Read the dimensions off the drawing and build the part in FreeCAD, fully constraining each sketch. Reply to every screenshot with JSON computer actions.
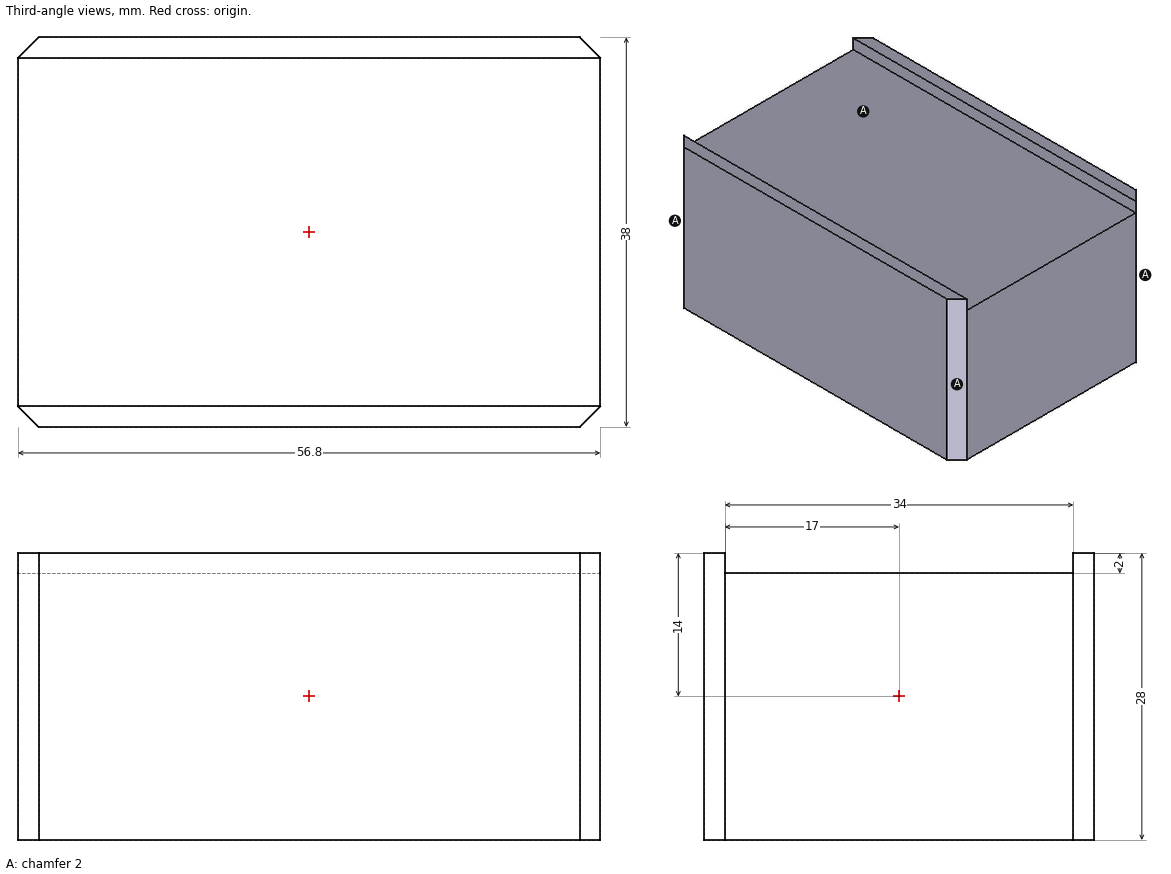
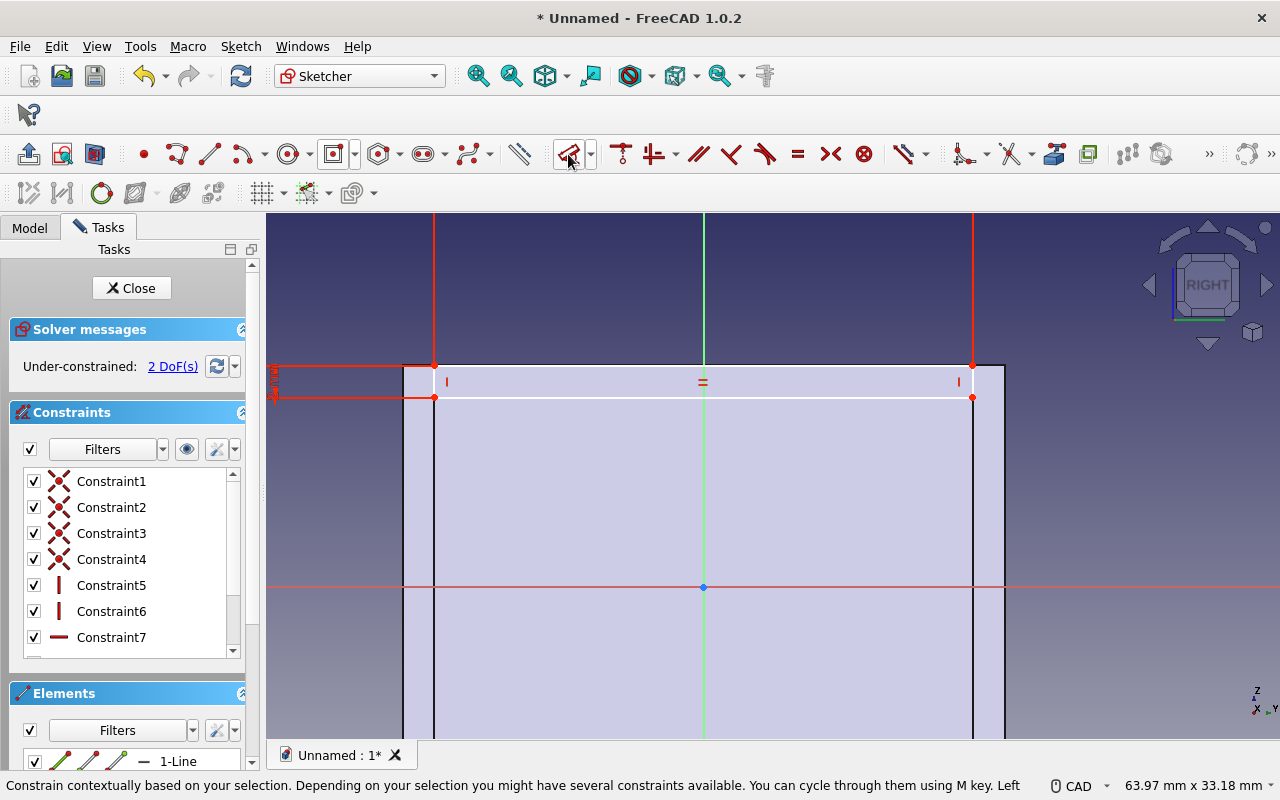
{"action": "left_click", "coordinate": [434, 366]}
{"action": "left_click", "coordinate": [569, 621]}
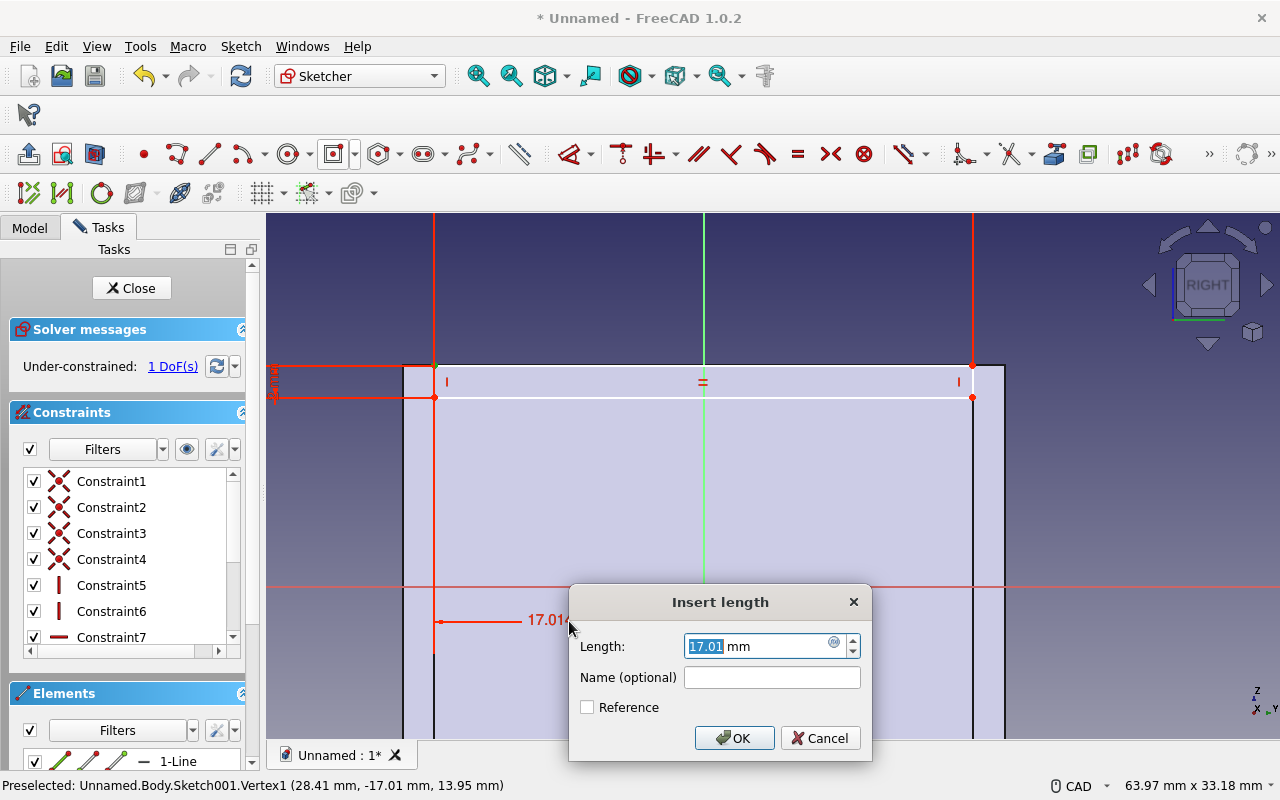
{"action": "type", "text": "17"}
{"action": "key", "text": "Return"}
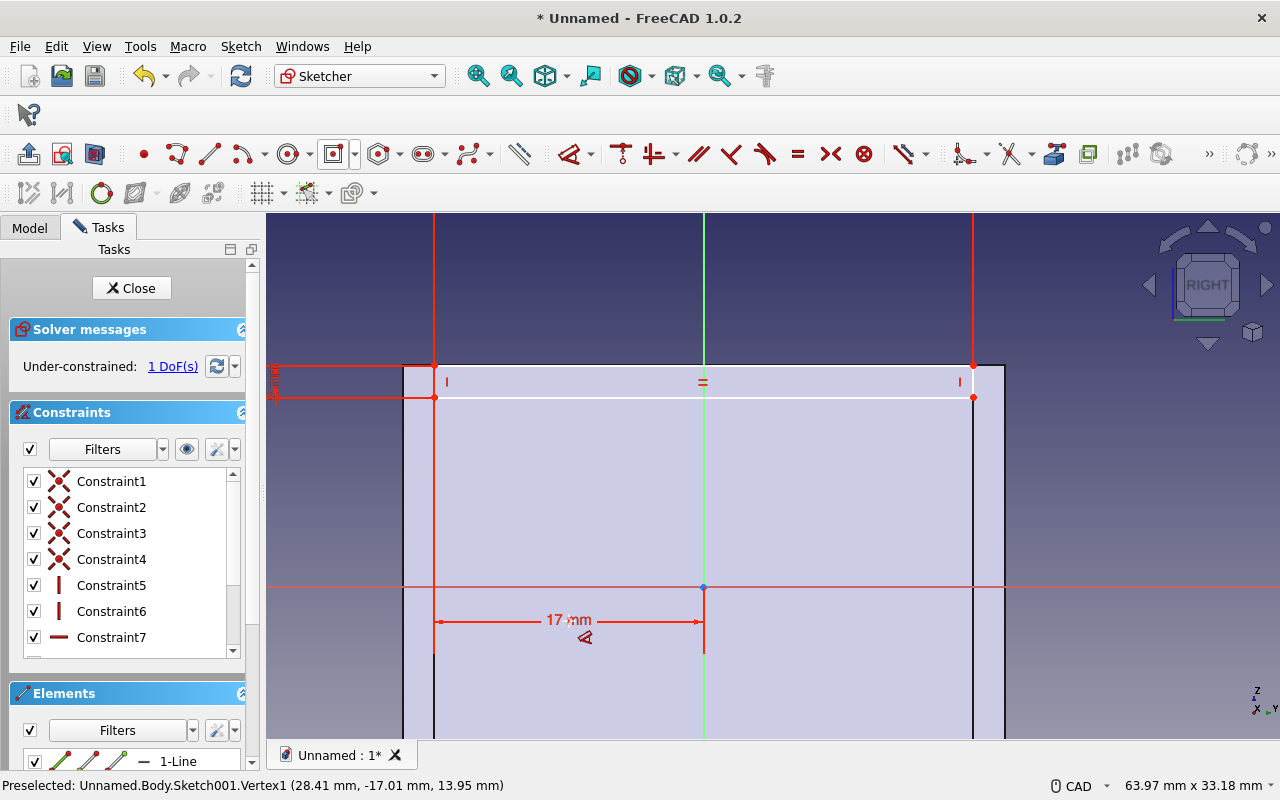
{"action": "left_click", "coordinate": [434, 366]}
{"action": "left_click", "coordinate": [400, 477]}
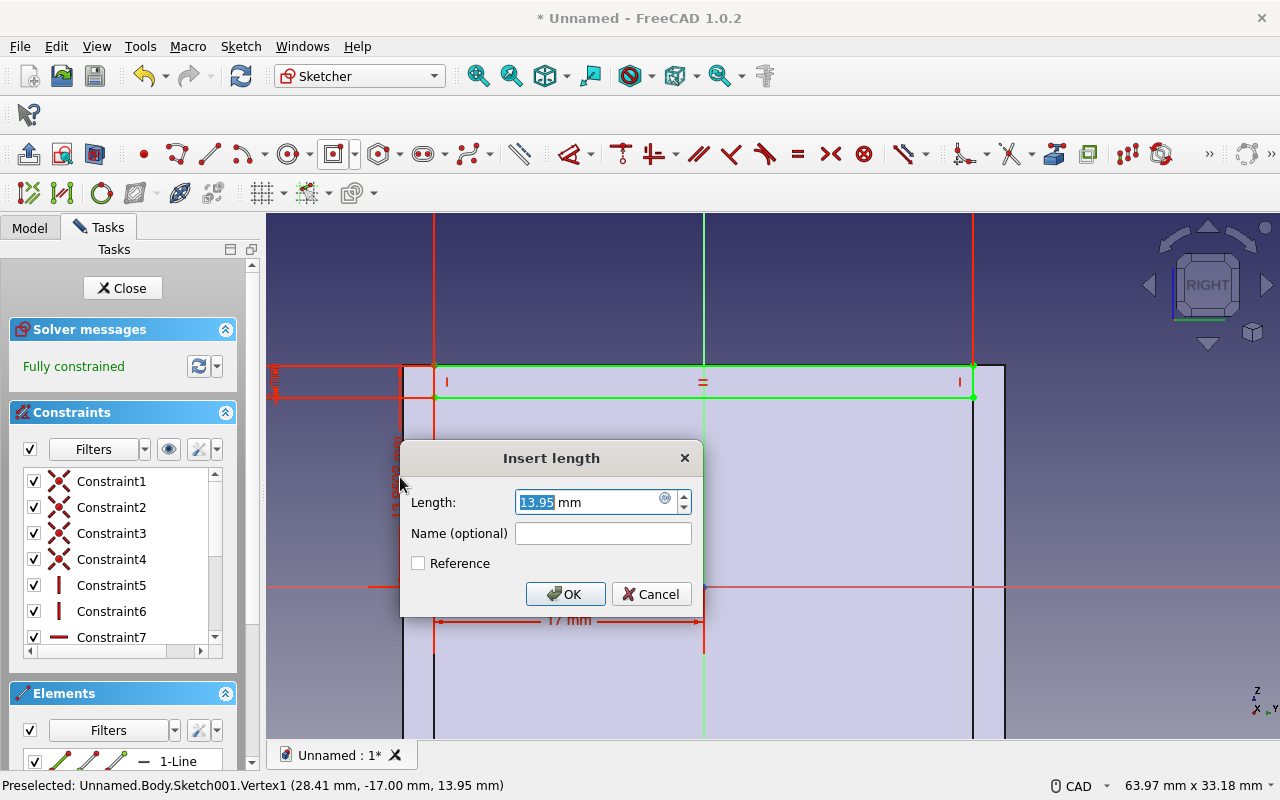
{"action": "type", "text": "14"}
{"action": "key", "text": "Return"}
{"action": "key", "text": "Escape"}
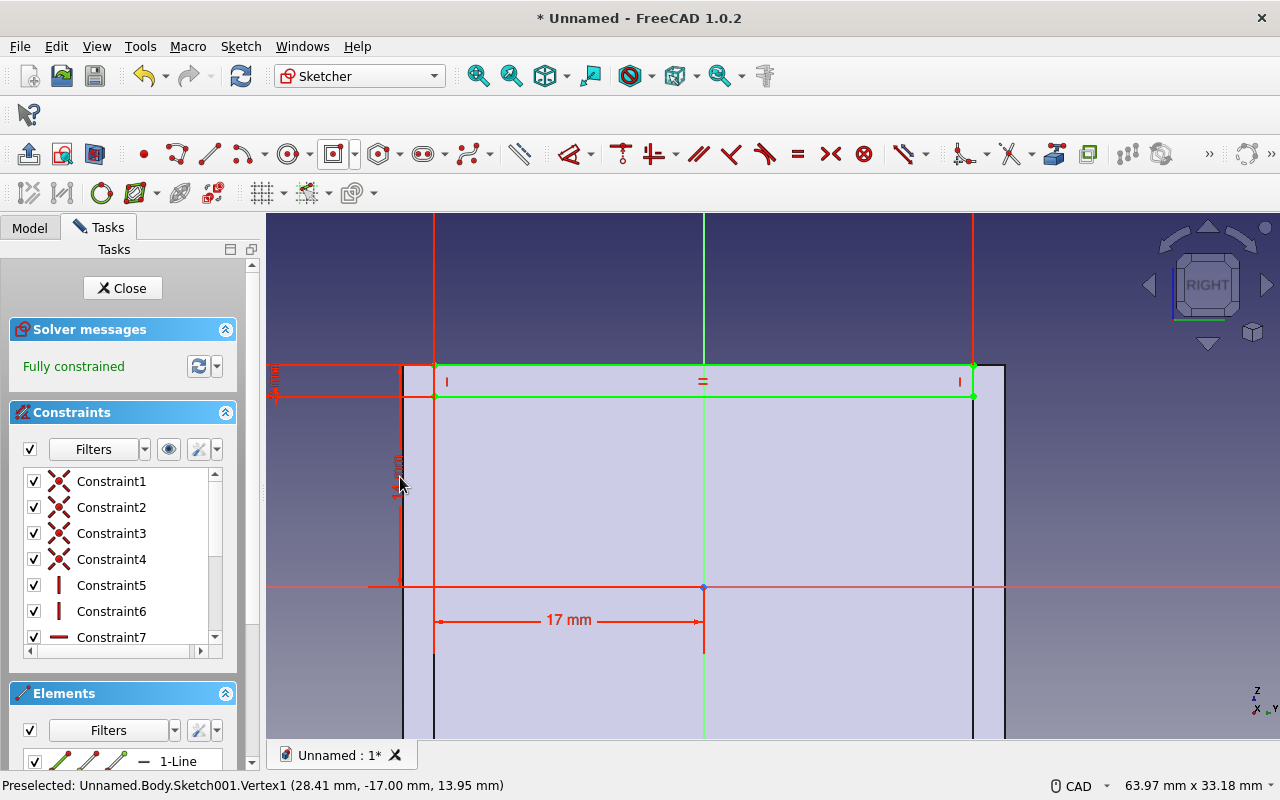
{"action": "left_click", "coordinate": [123, 288]}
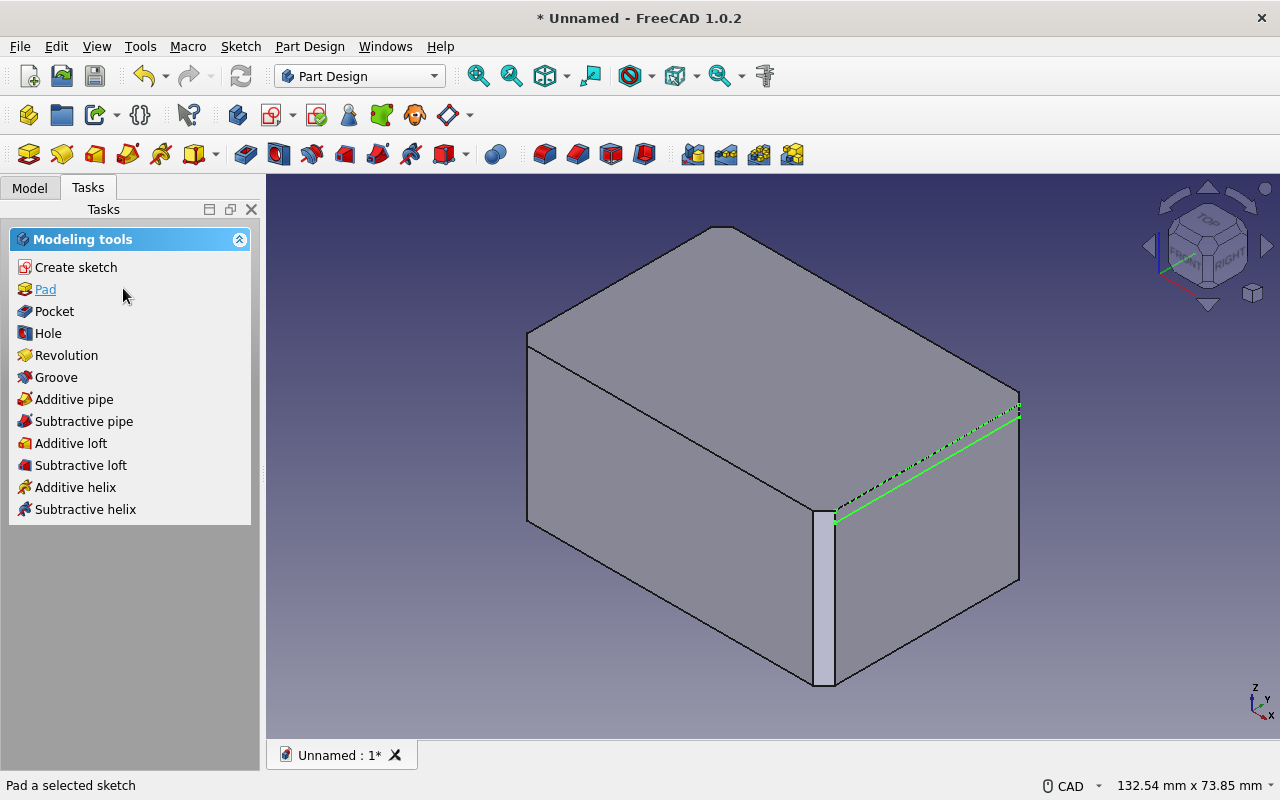
{"action": "left_click", "coordinate": [246, 154]}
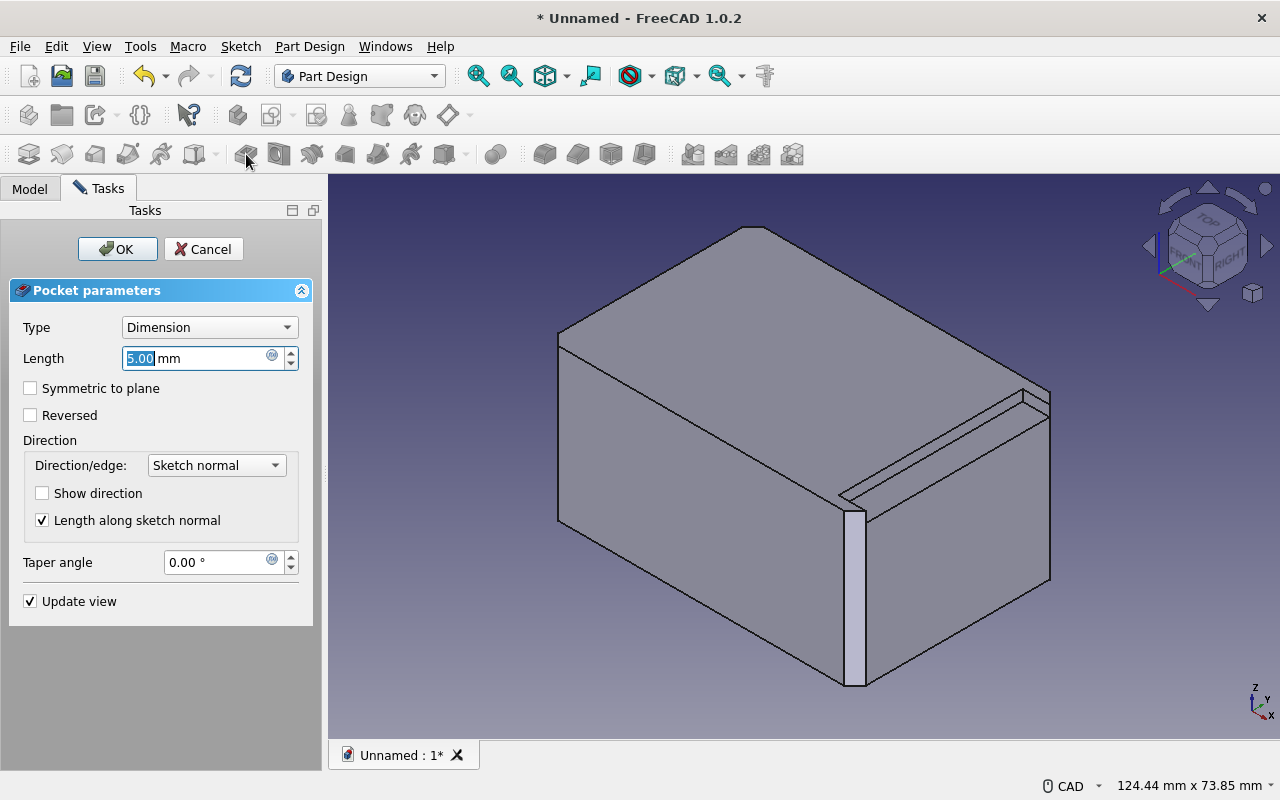
{"action": "left_click", "coordinate": [210, 328]}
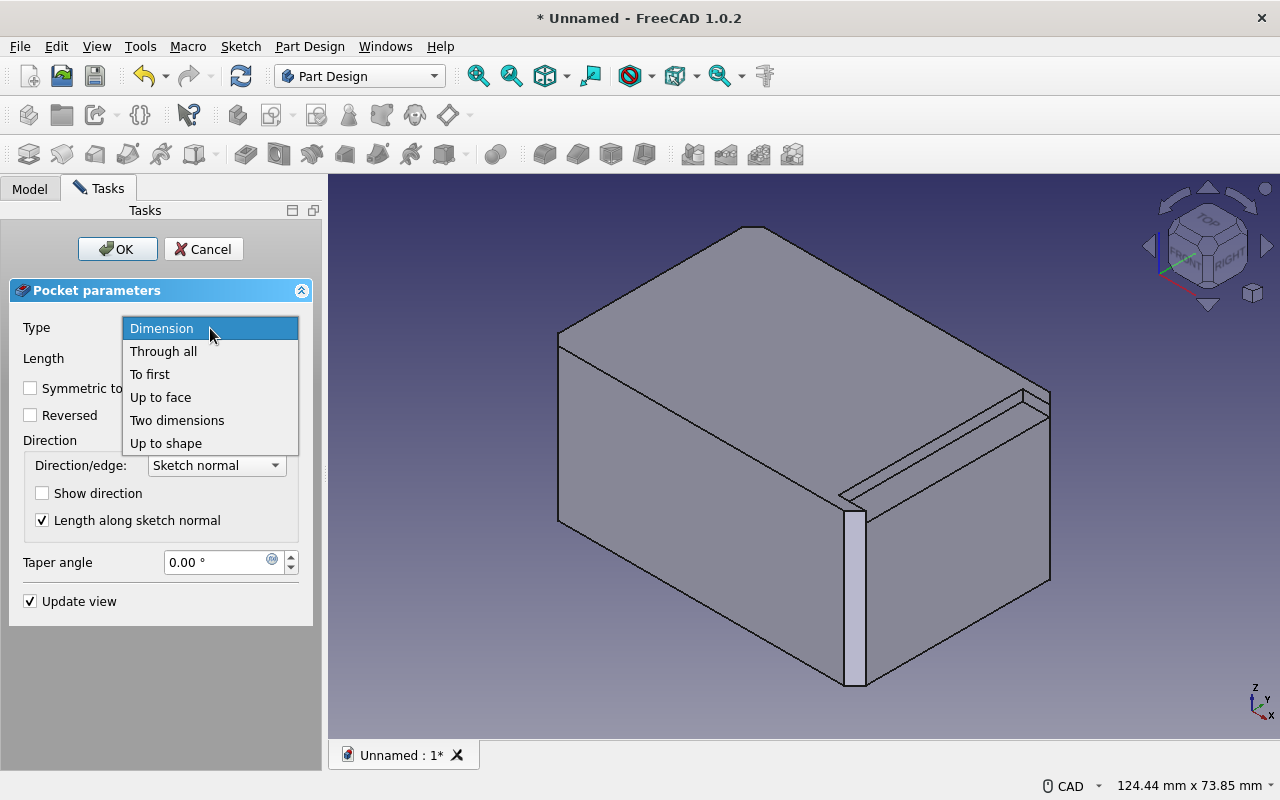
{"action": "left_click", "coordinate": [208, 352]}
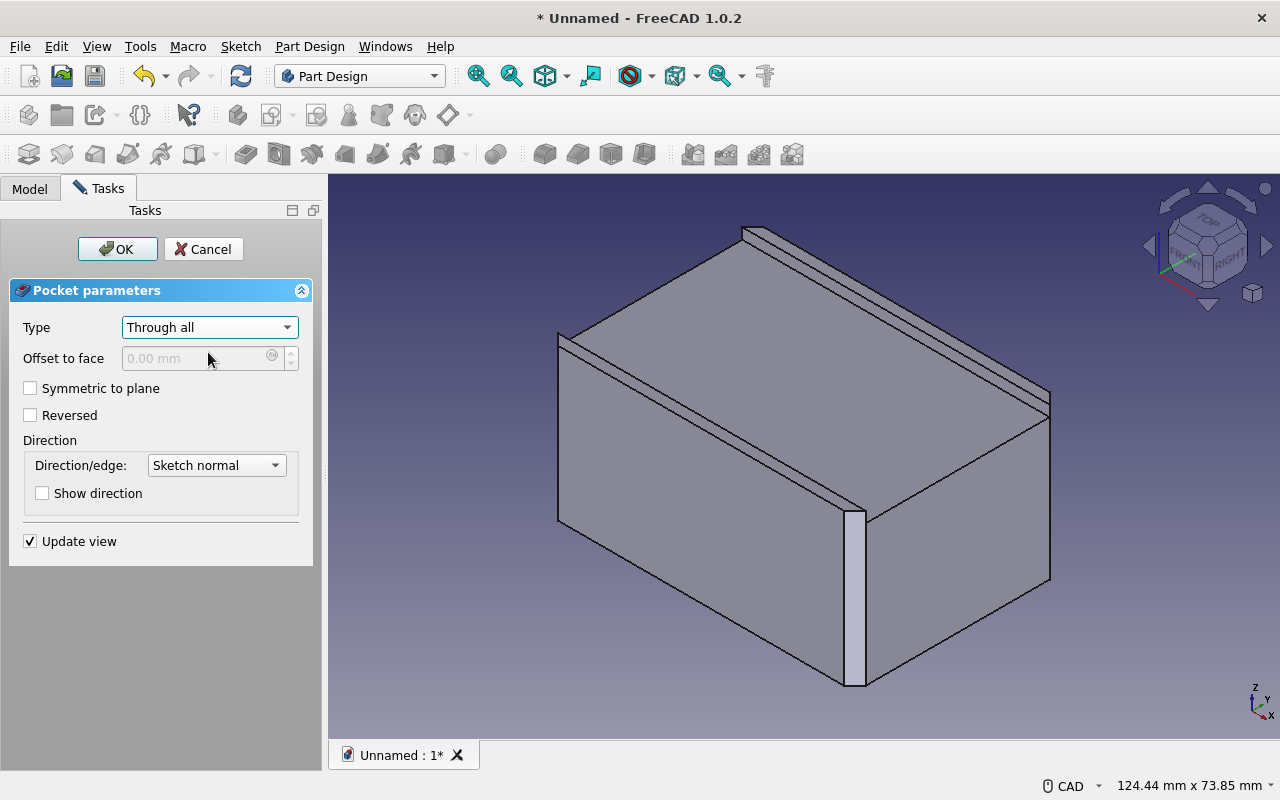
{"action": "left_click", "coordinate": [118, 249]}